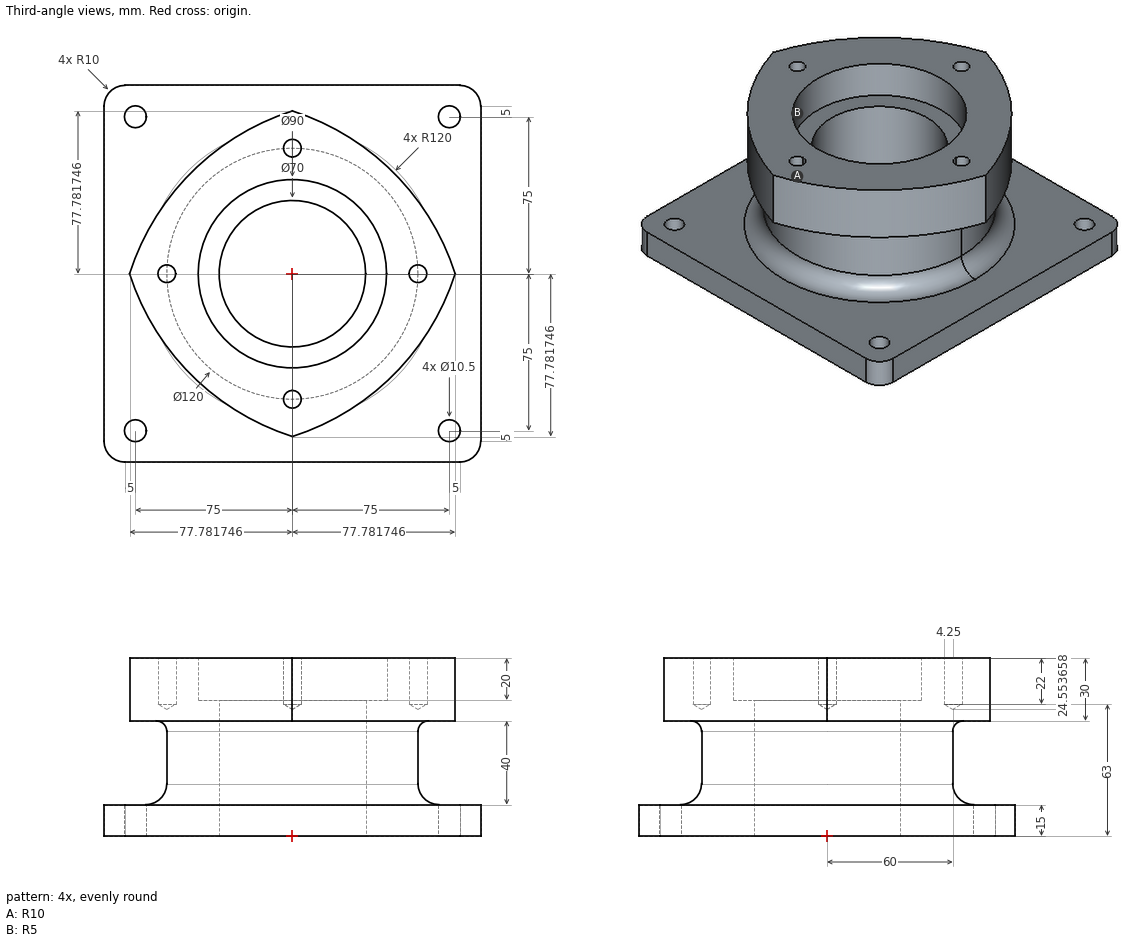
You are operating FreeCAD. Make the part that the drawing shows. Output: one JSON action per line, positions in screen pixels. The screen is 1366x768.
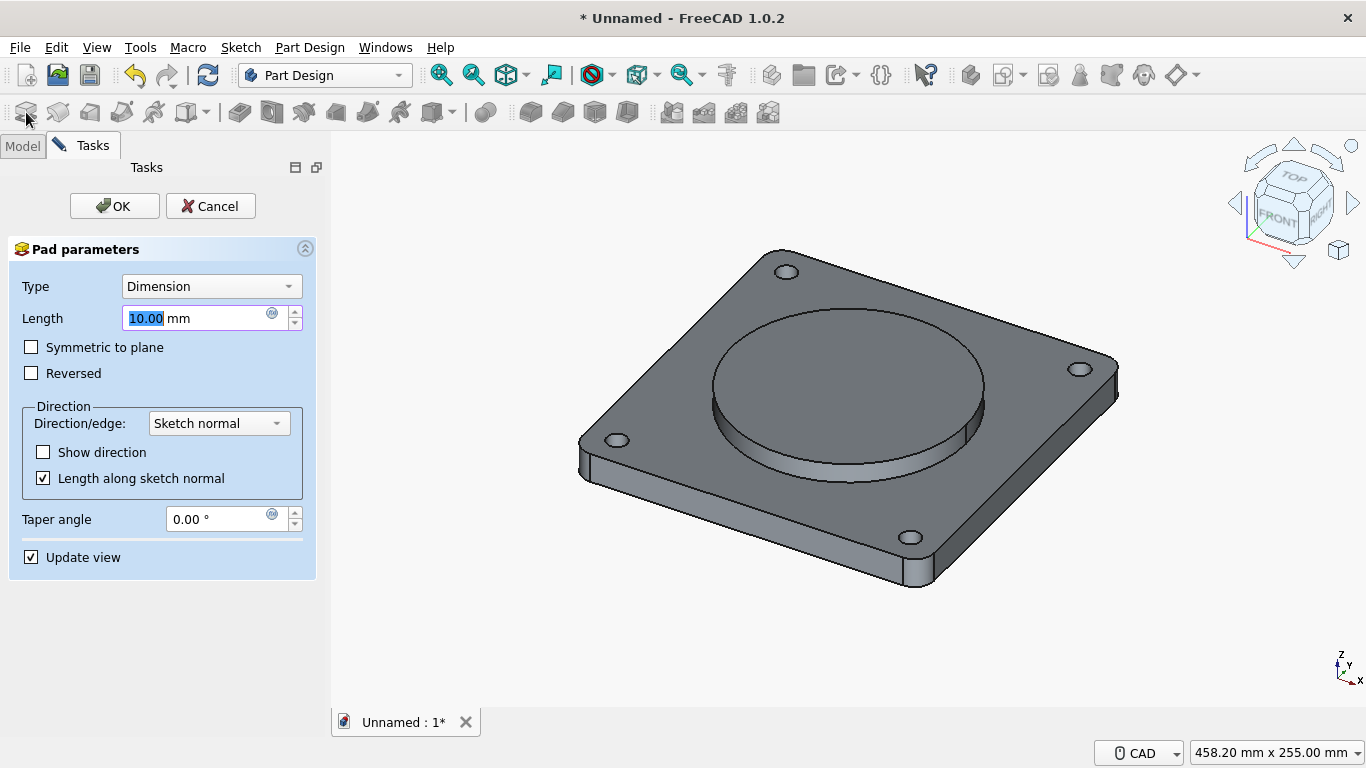
{"action": "type", "text": "40"}
{"action": "key", "text": "Tab"}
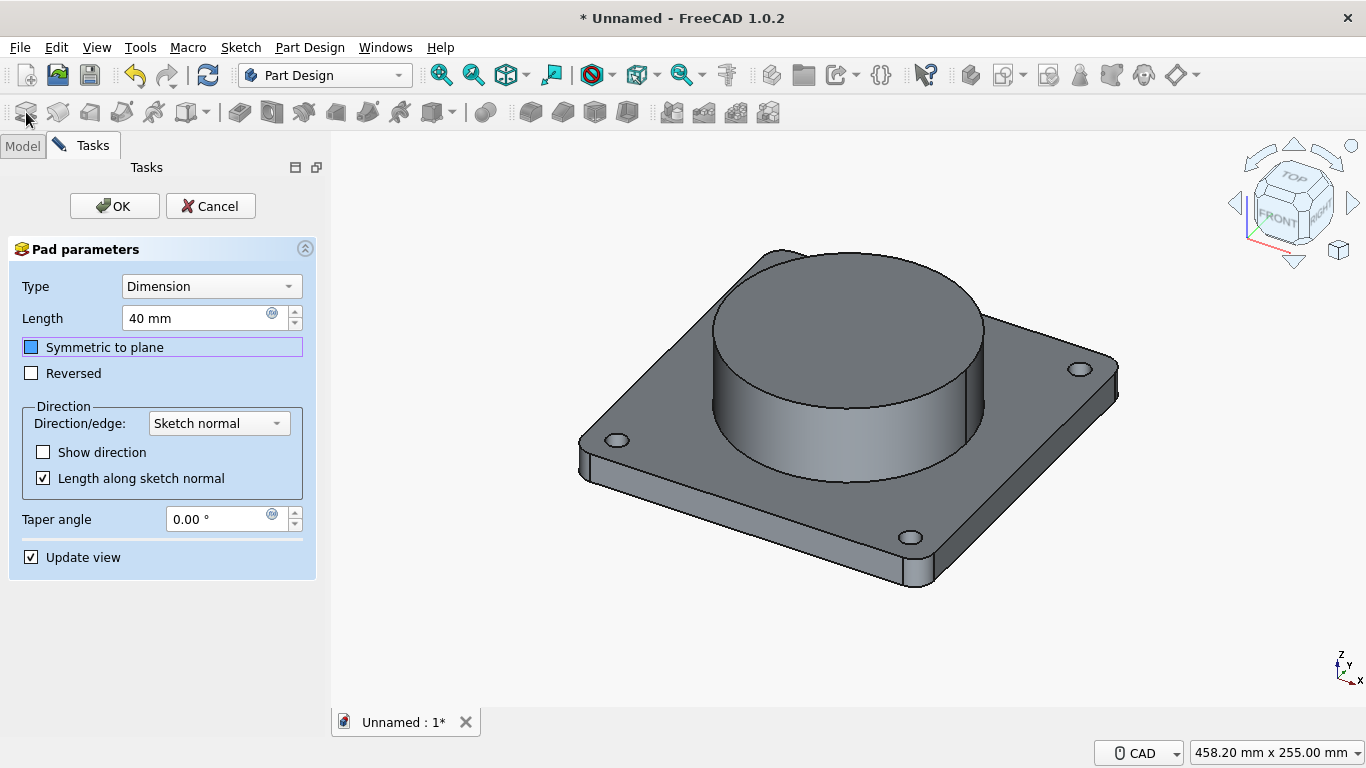
{"action": "left_click", "coordinate": [115, 206]}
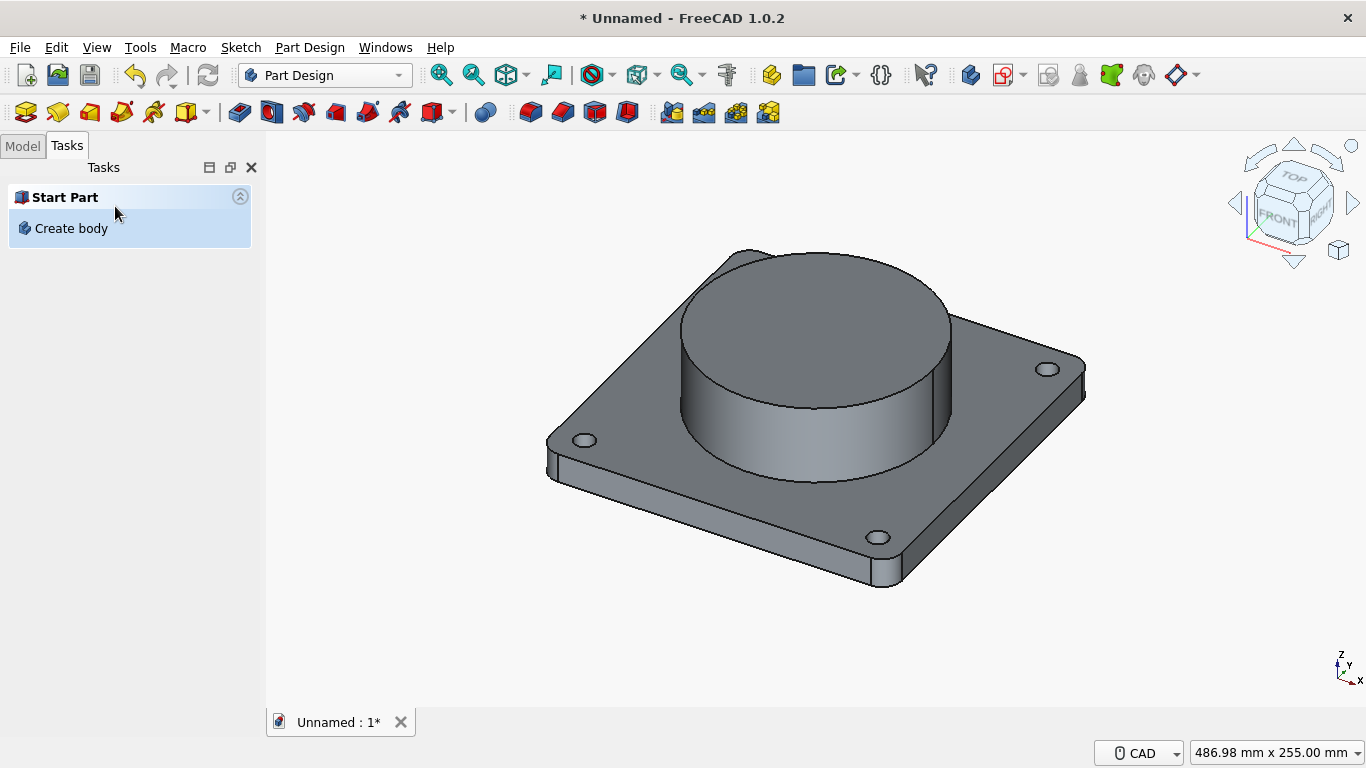
{"action": "left_click", "coordinate": [816, 330]}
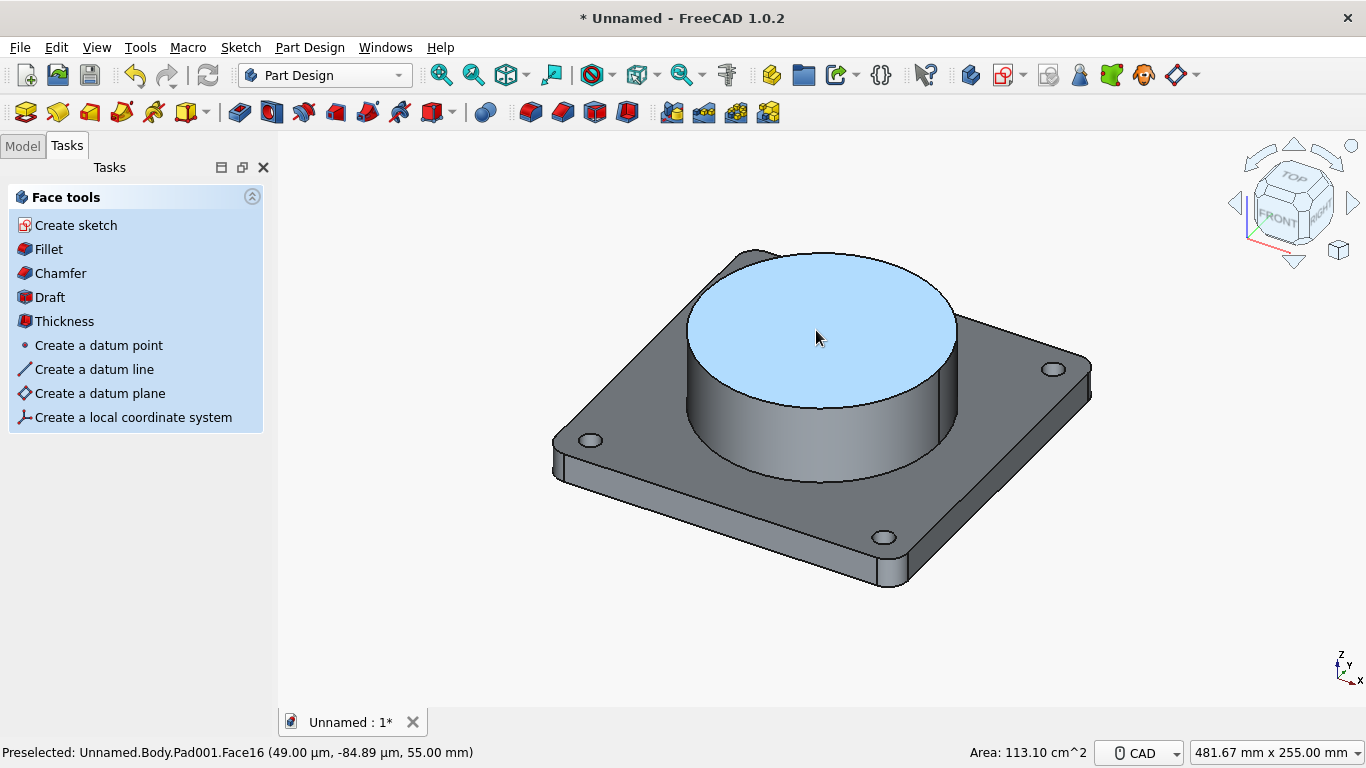
{"action": "left_click", "coordinate": [1004, 76]}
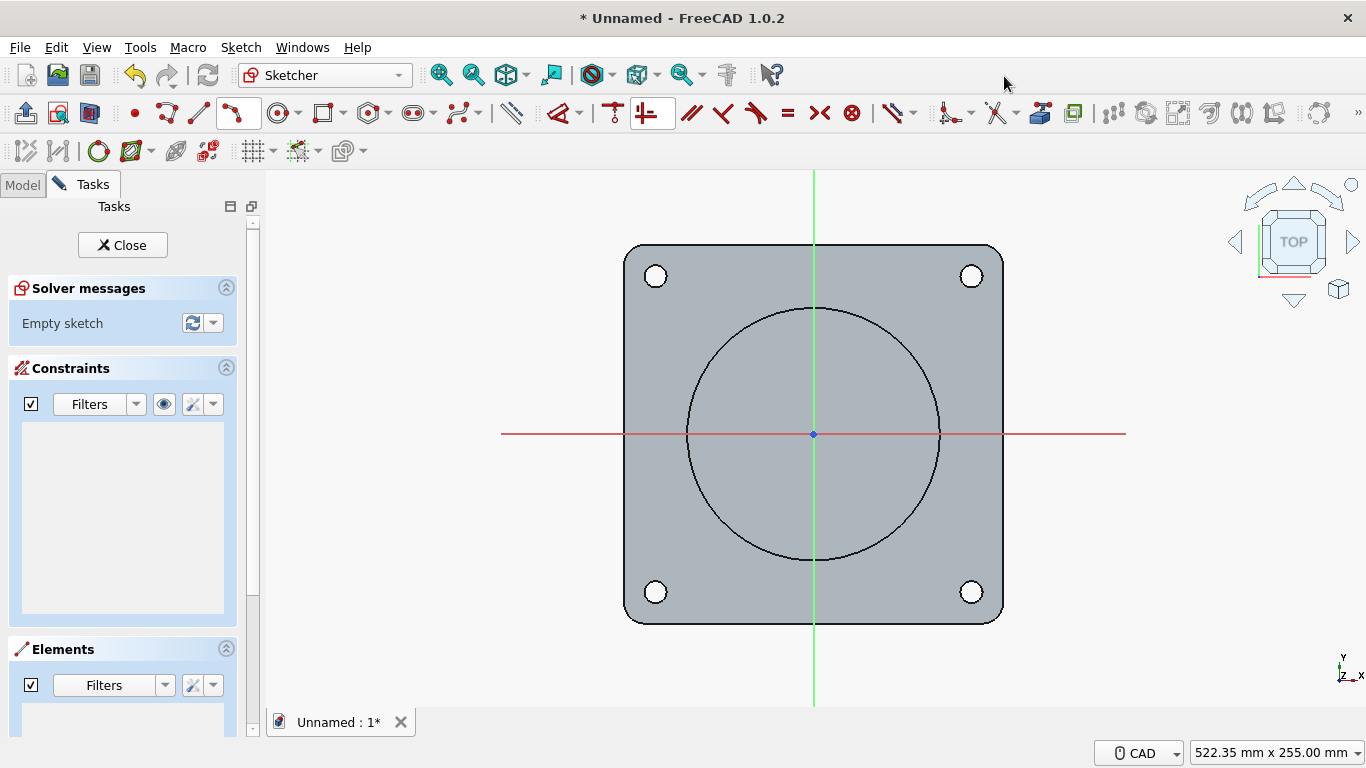
{"action": "left_click", "coordinate": [232, 114]}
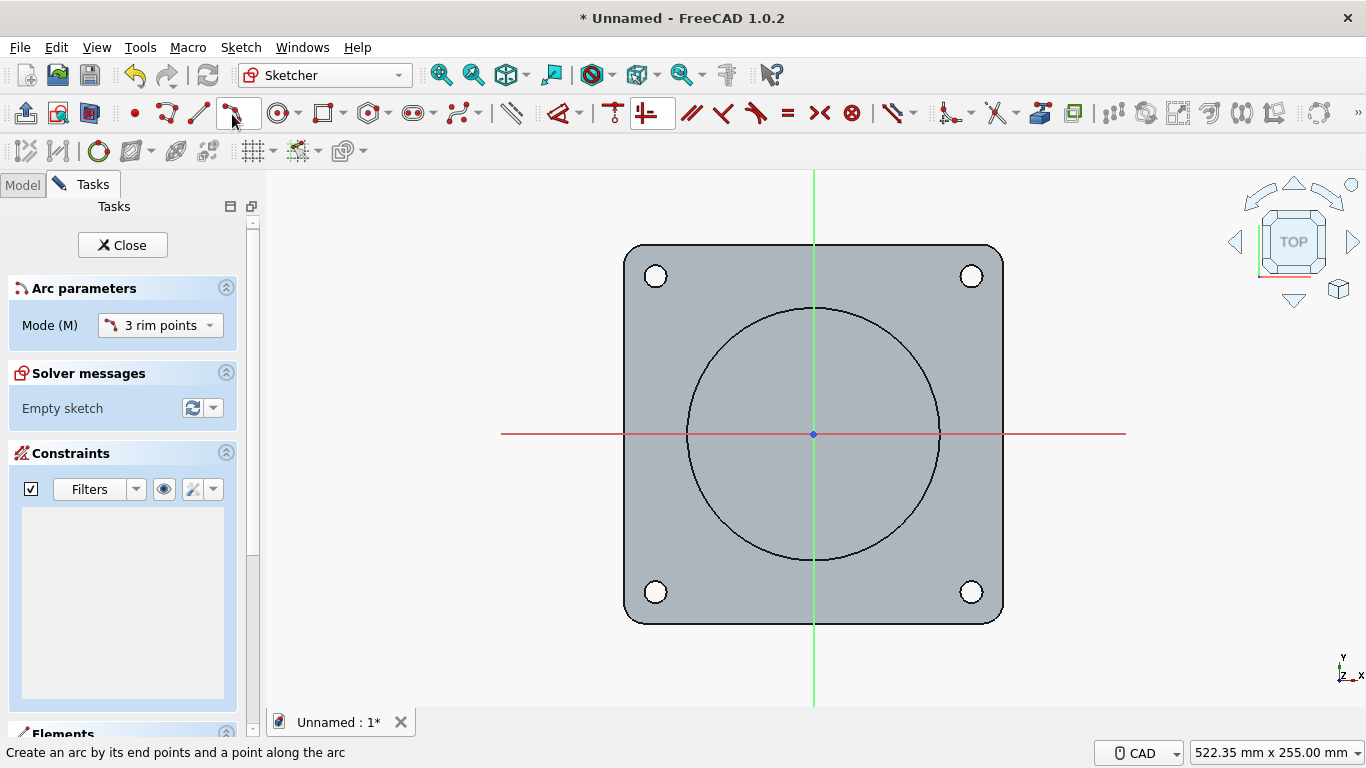
{"action": "left_click", "coordinate": [977, 434]}
{"action": "left_click", "coordinate": [814, 270]}
{"action": "left_click", "coordinate": [915, 332]}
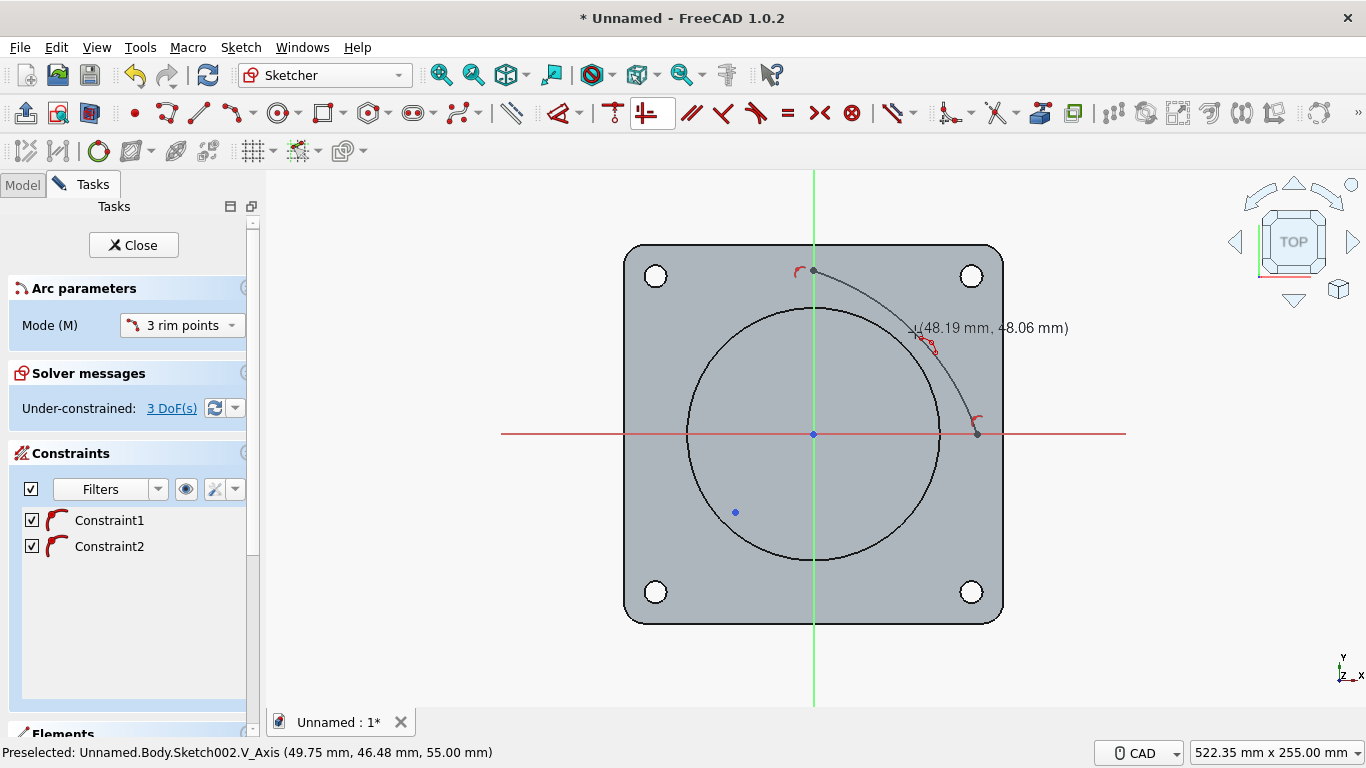
{"action": "left_click", "coordinate": [814, 271]}
{"action": "left_click", "coordinate": [650, 434]}
{"action": "left_click", "coordinate": [712, 332]}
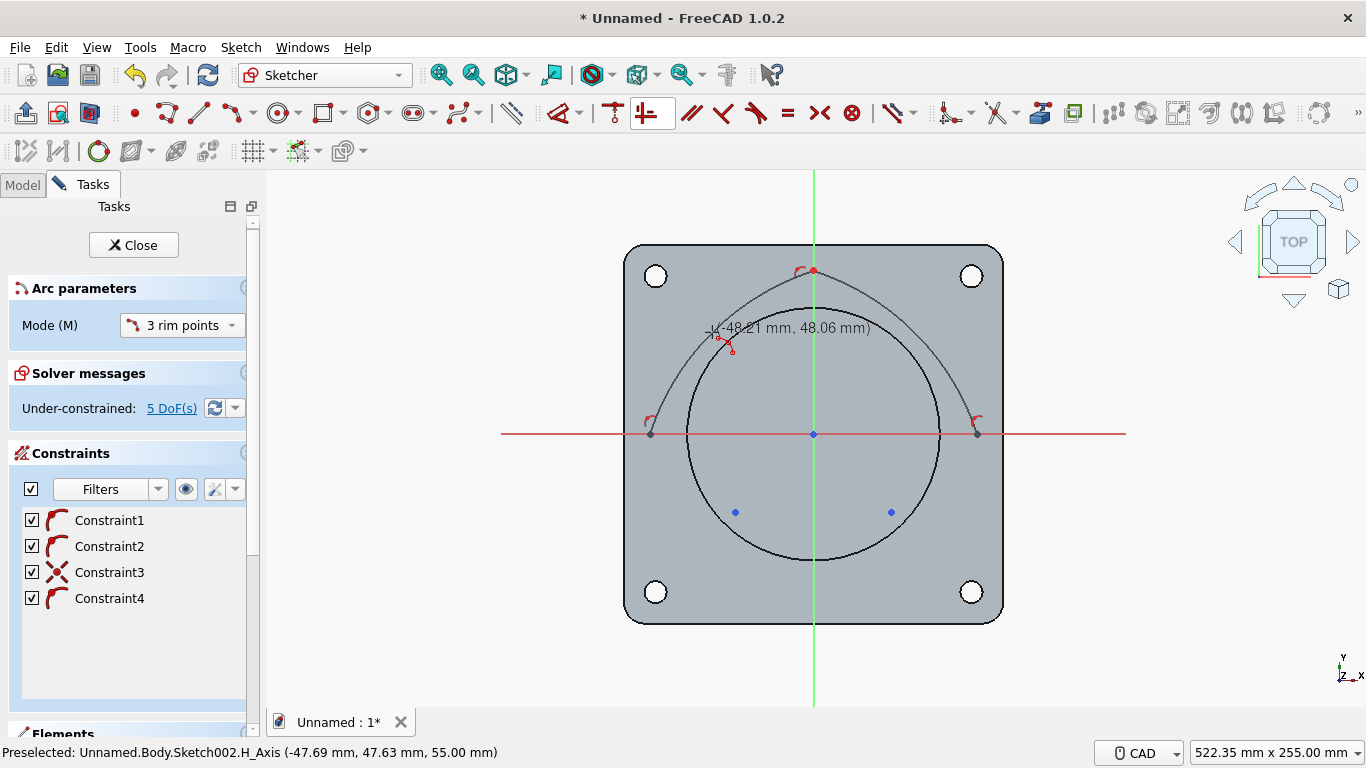
{"action": "left_click", "coordinate": [650, 434]}
{"action": "left_click", "coordinate": [814, 598]}
{"action": "left_click", "coordinate": [712, 536]}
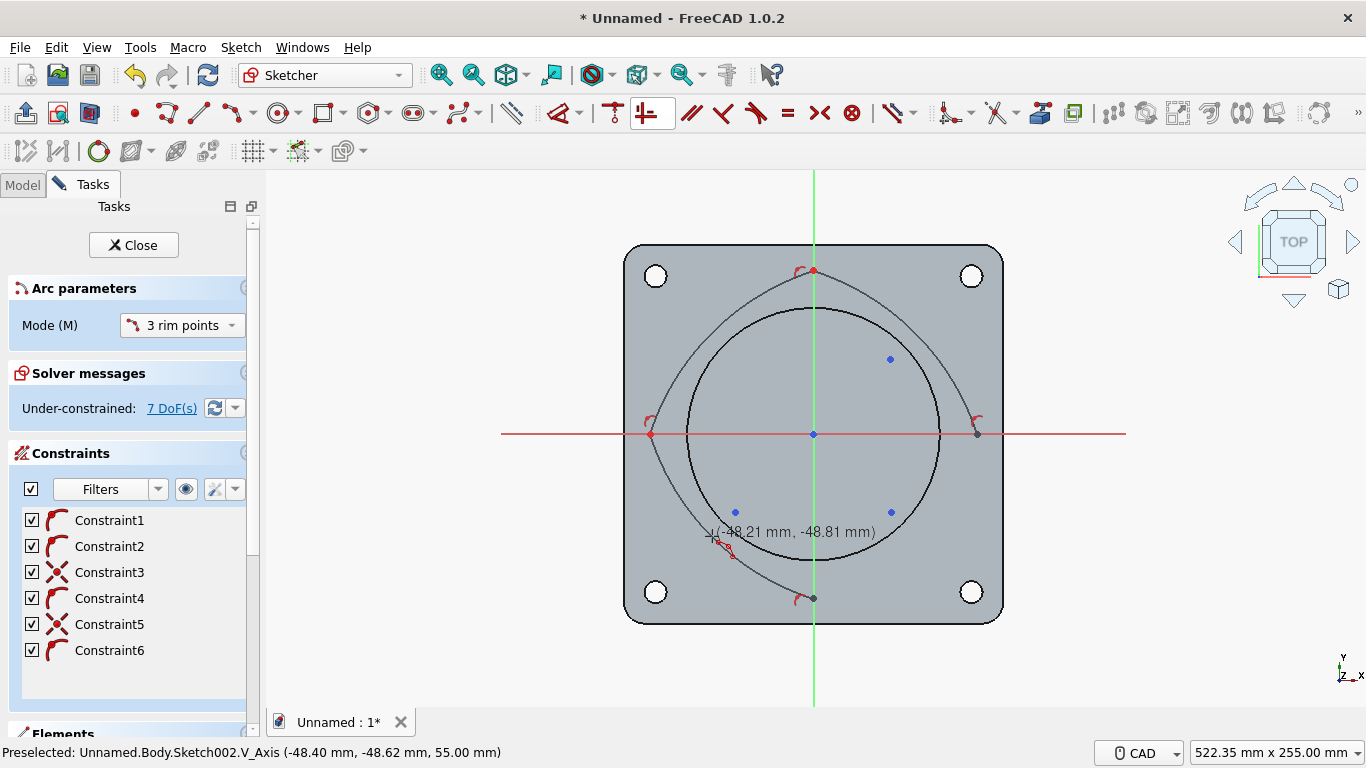
{"action": "left_click", "coordinate": [814, 599]}
{"action": "left_click", "coordinate": [977, 434]}
{"action": "left_click", "coordinate": [915, 536]}
{"action": "key", "text": "Escape"}